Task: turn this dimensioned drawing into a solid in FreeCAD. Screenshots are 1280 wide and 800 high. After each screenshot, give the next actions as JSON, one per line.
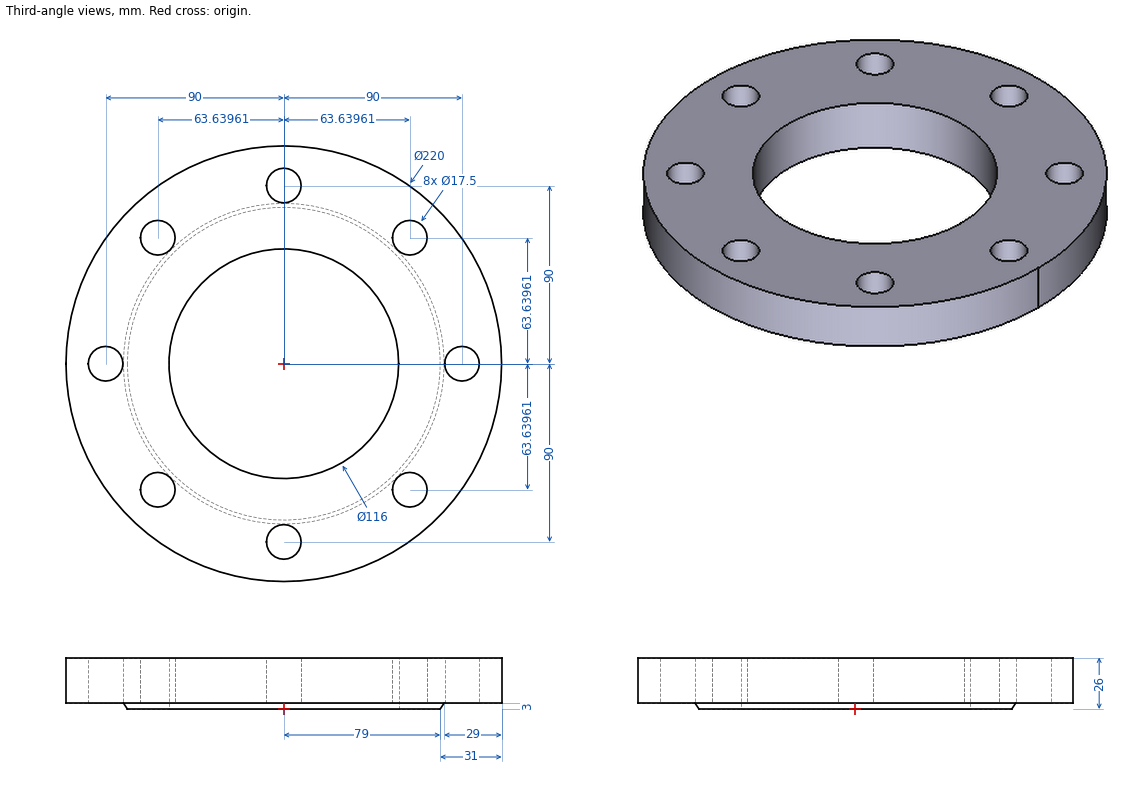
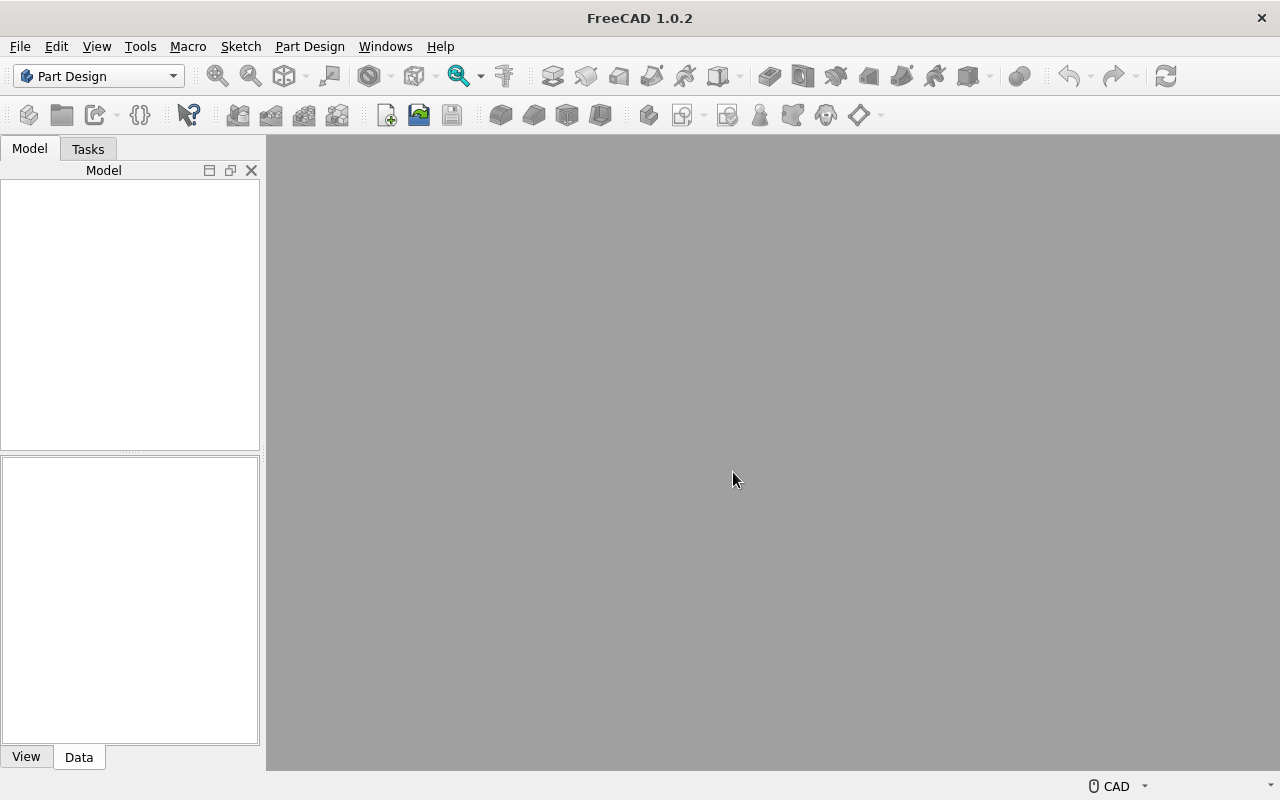
{"action": "left_click", "coordinate": [386, 116]}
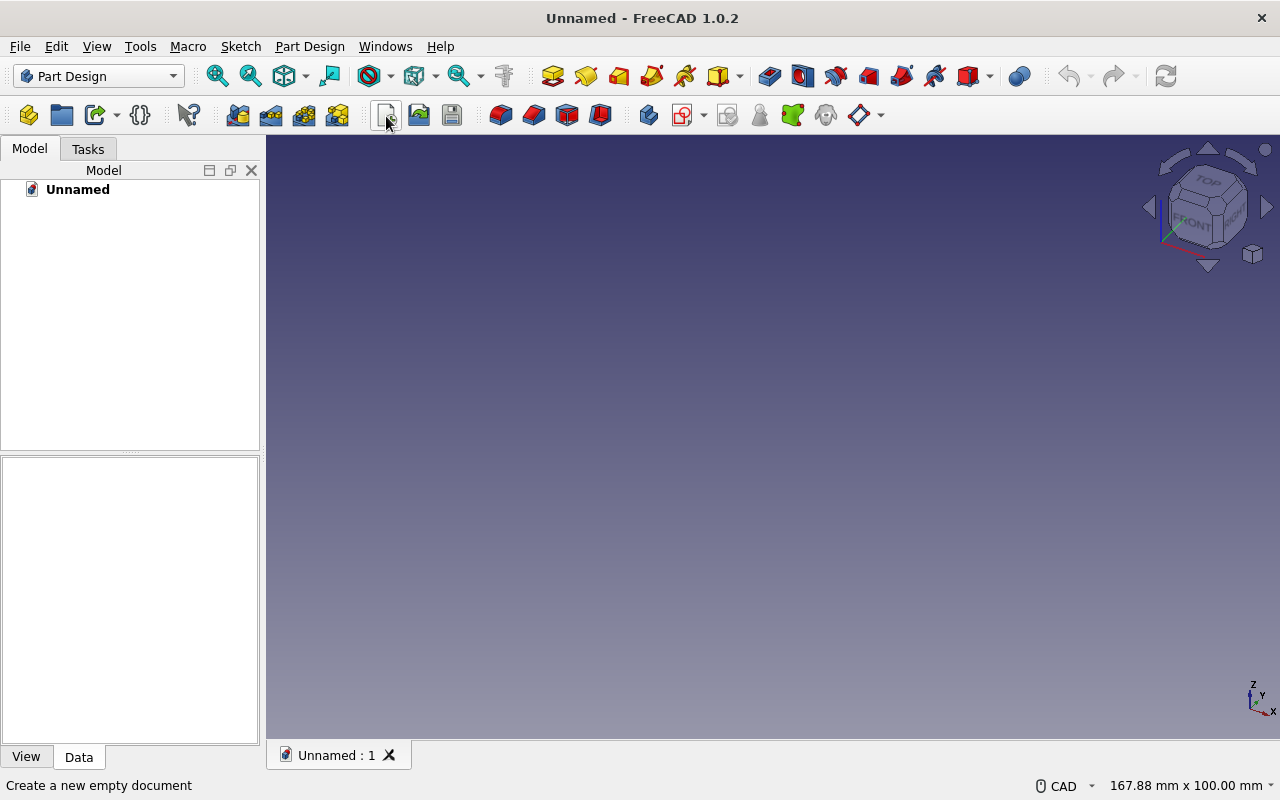
{"action": "left_click", "coordinate": [682, 116]}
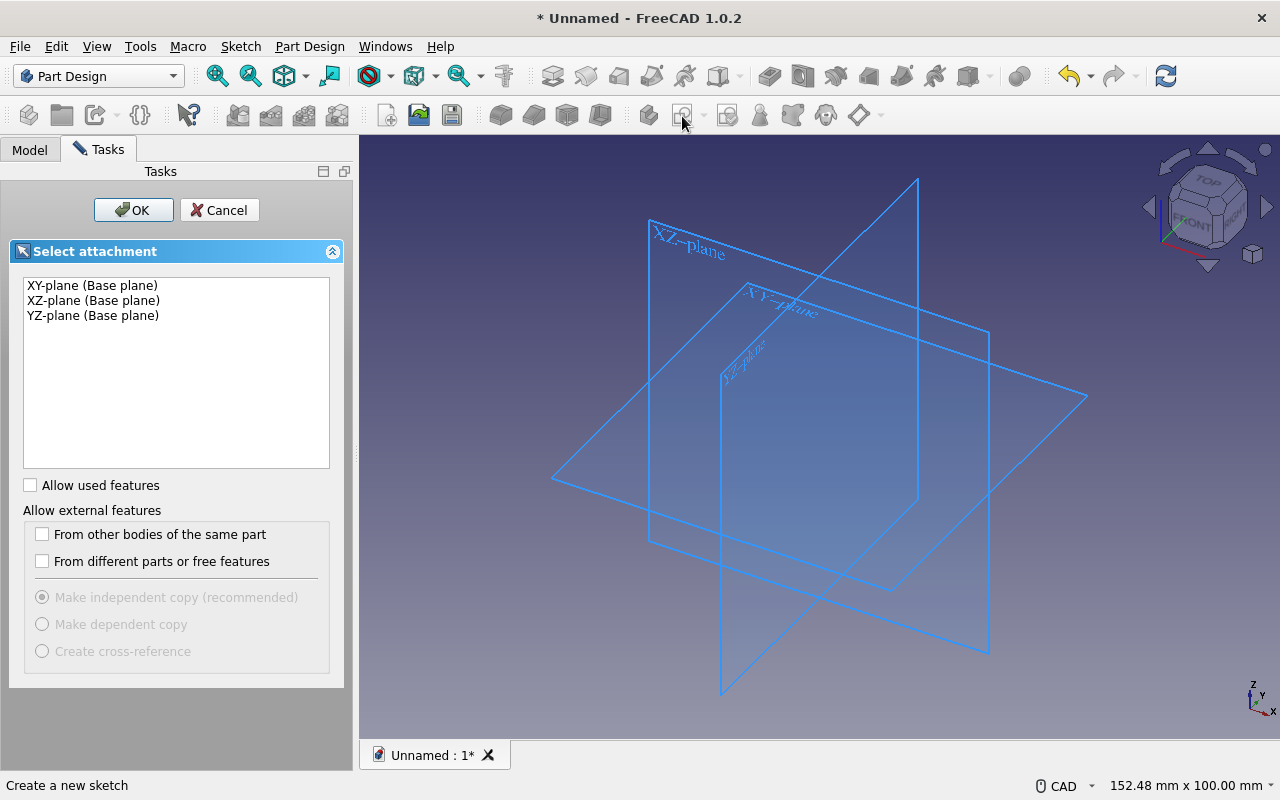
{"action": "left_click", "coordinate": [84, 286]}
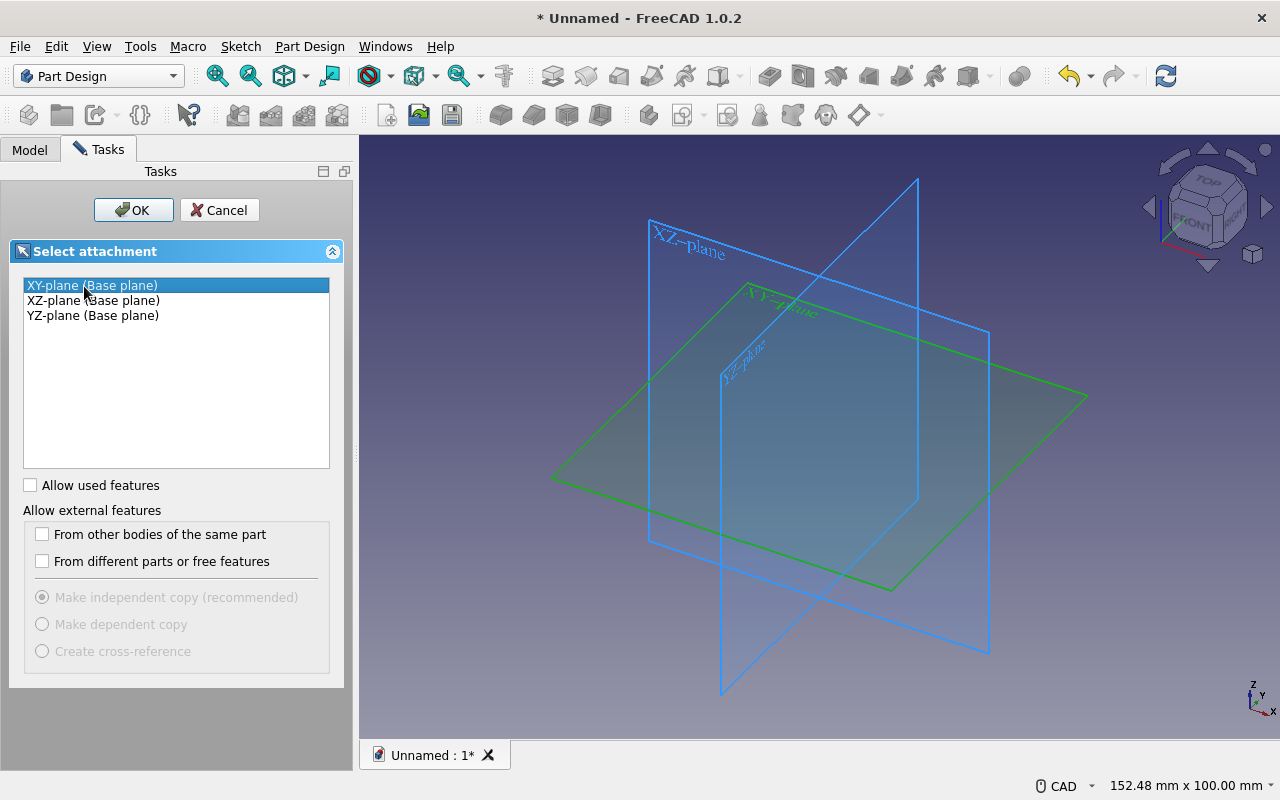
{"action": "left_click", "coordinate": [134, 210]}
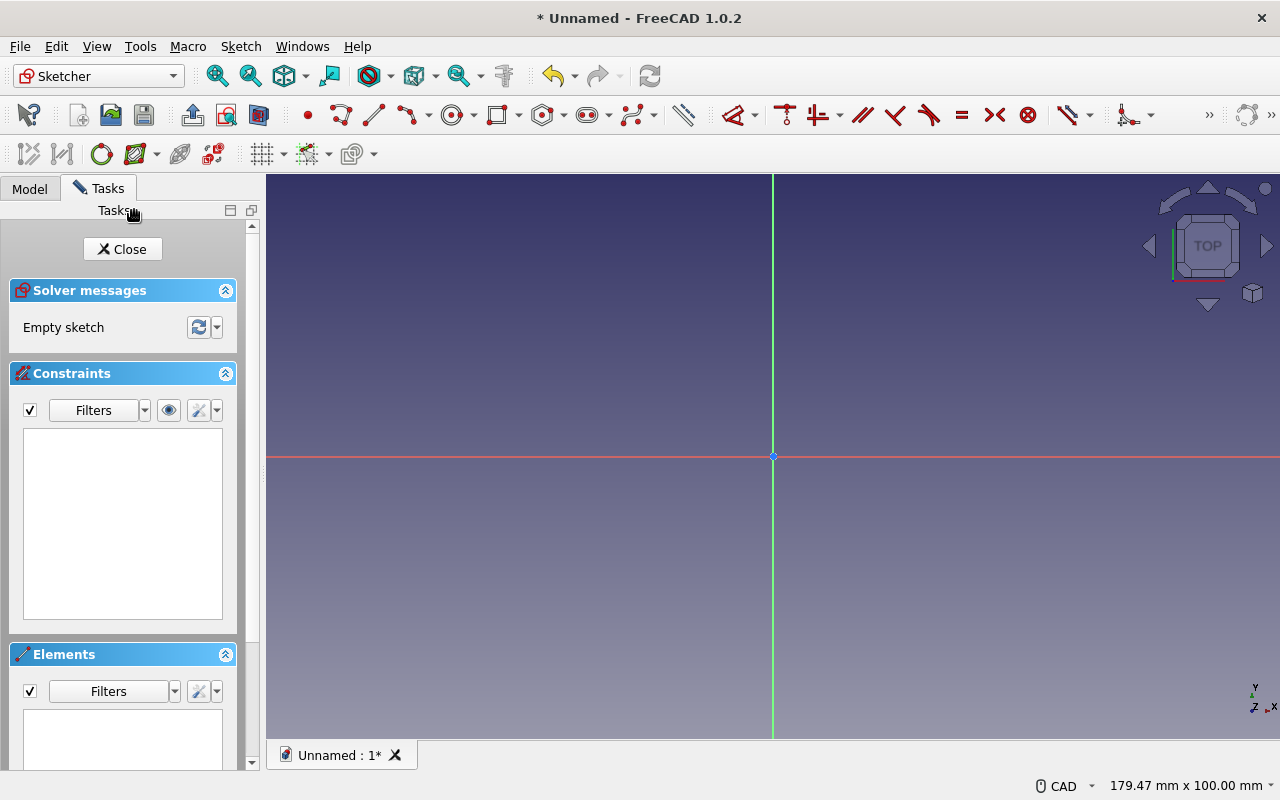
{"action": "scroll", "coordinate": [675, 456], "scroll_direction": "down", "scroll_amount": 6}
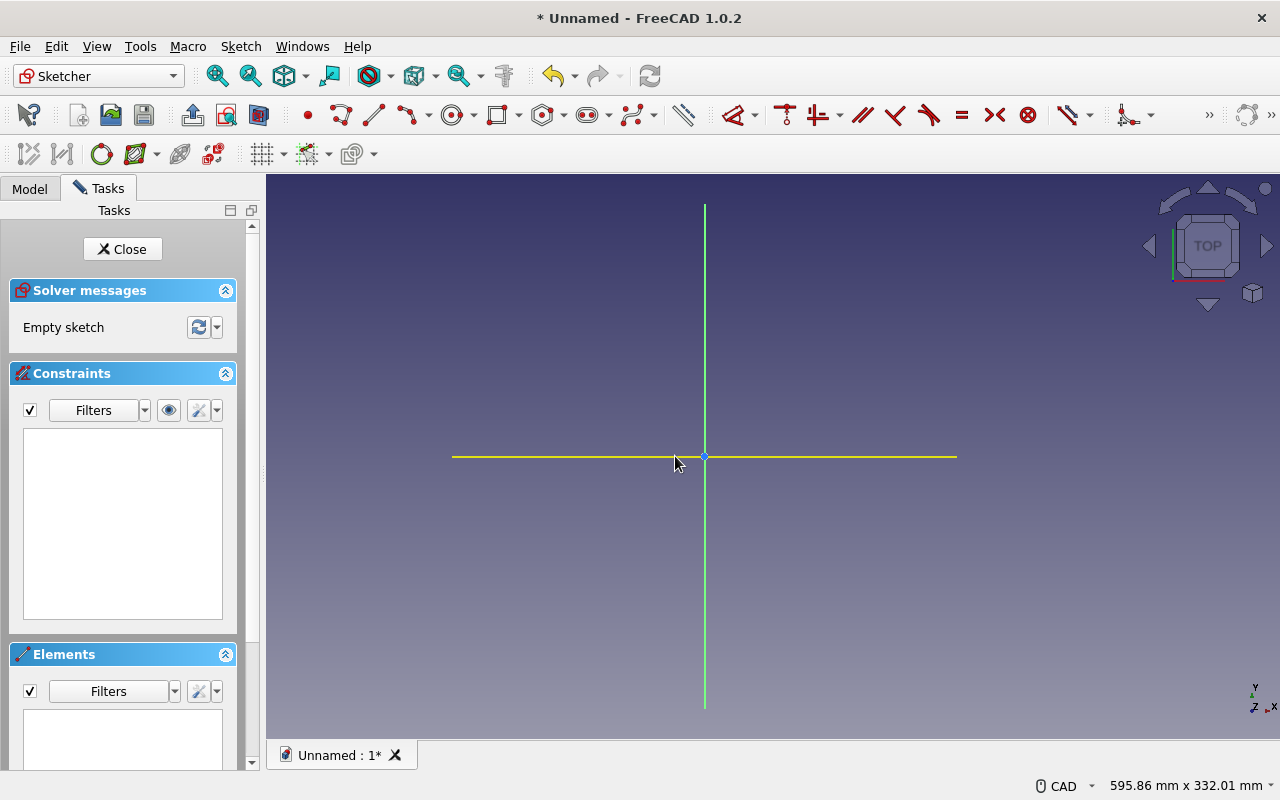
{"action": "left_click", "coordinate": [452, 116]}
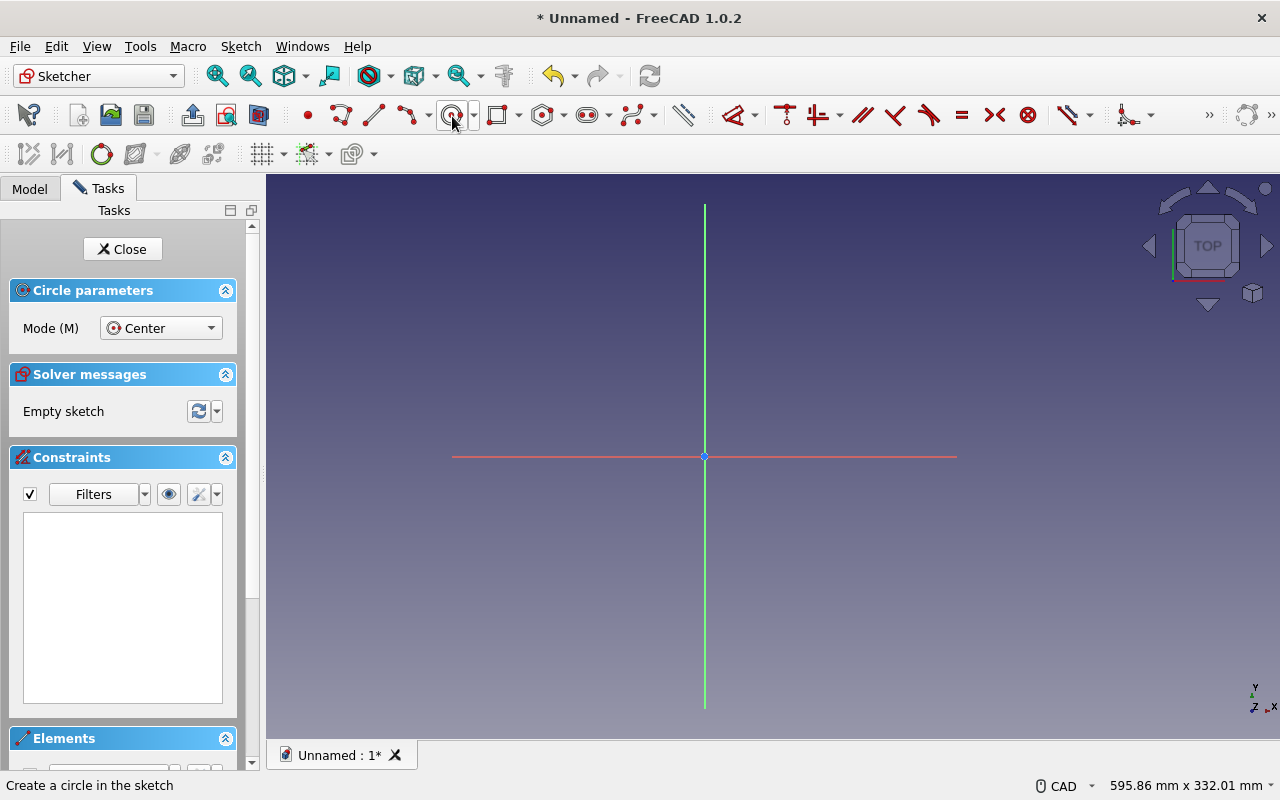
{"action": "left_click", "coordinate": [705, 456]}
{"action": "left_click", "coordinate": [837, 324]}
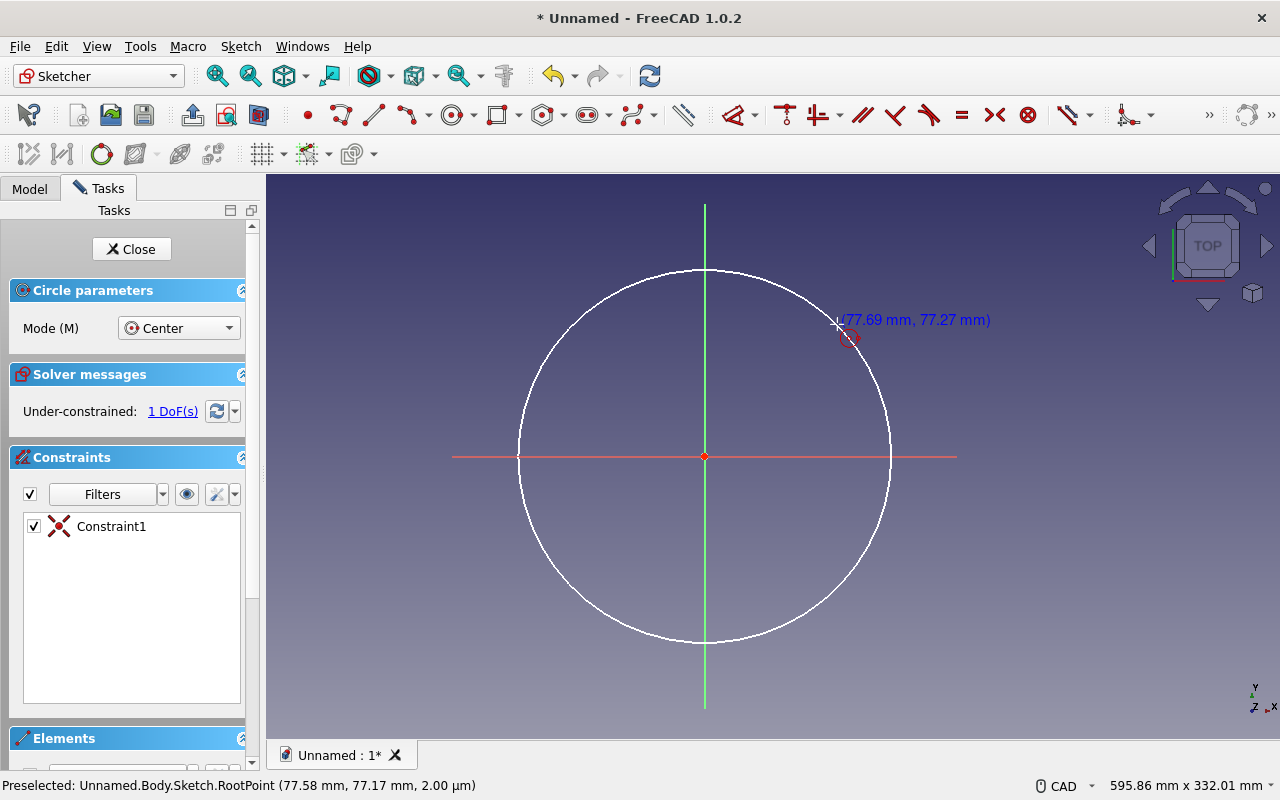
{"action": "scroll", "coordinate": [813, 348], "scroll_direction": "up", "scroll_amount": 3}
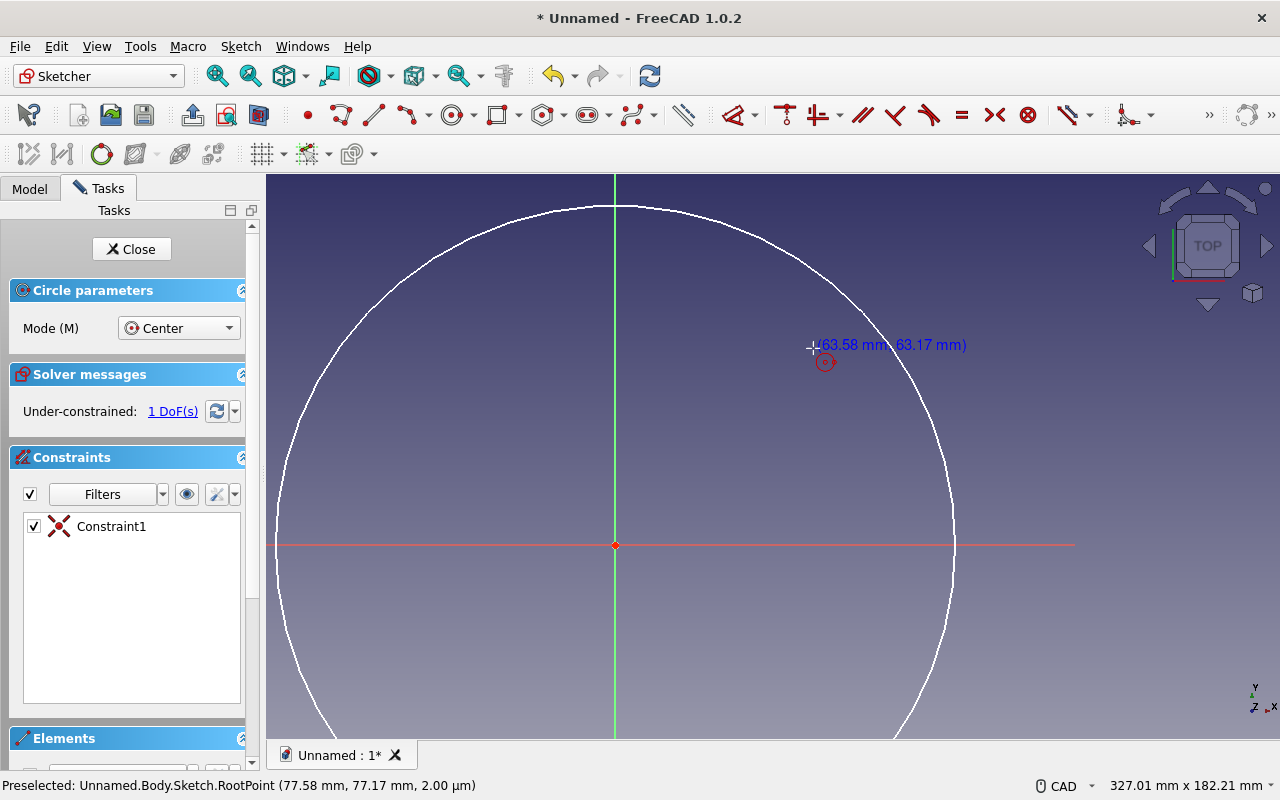
{"action": "left_click", "coordinate": [813, 348]}
{"action": "left_click", "coordinate": [832, 329]}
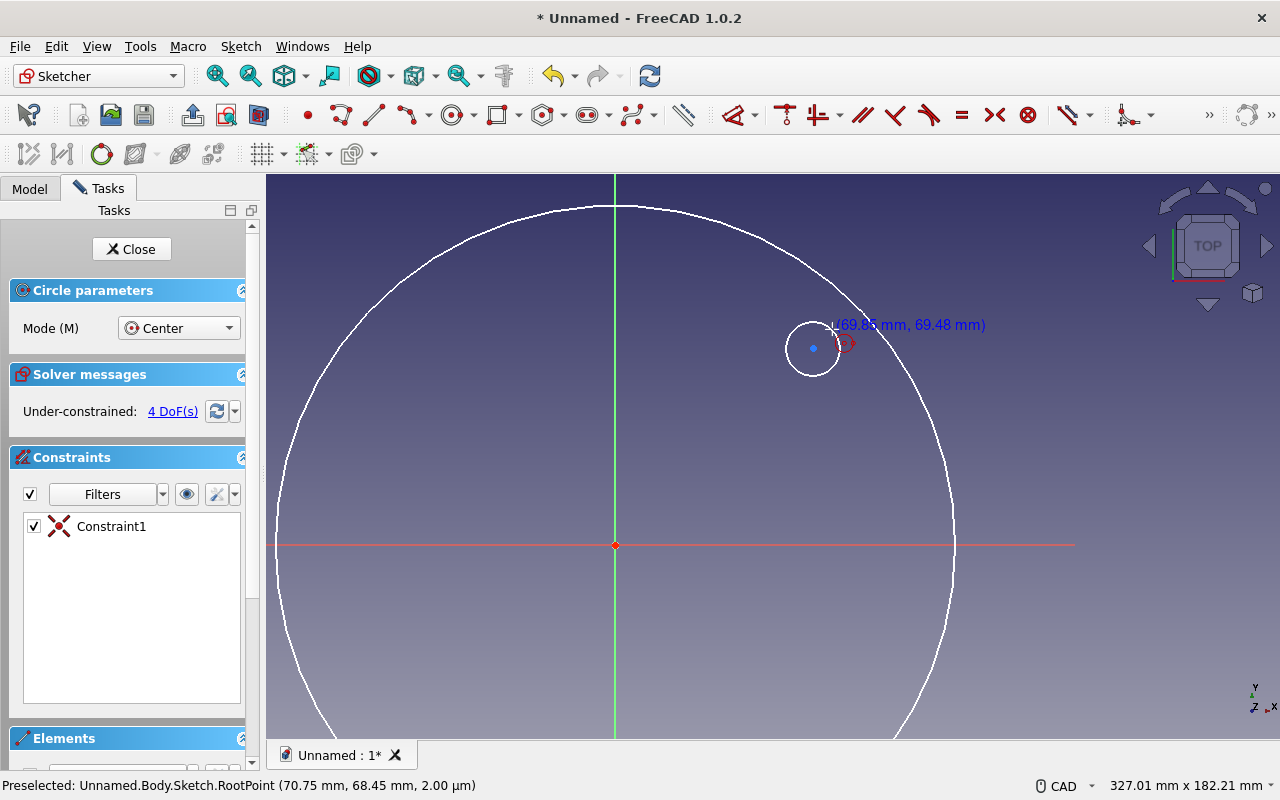
{"action": "left_click", "coordinate": [615, 266]}
{"action": "left_click", "coordinate": [635, 247]}